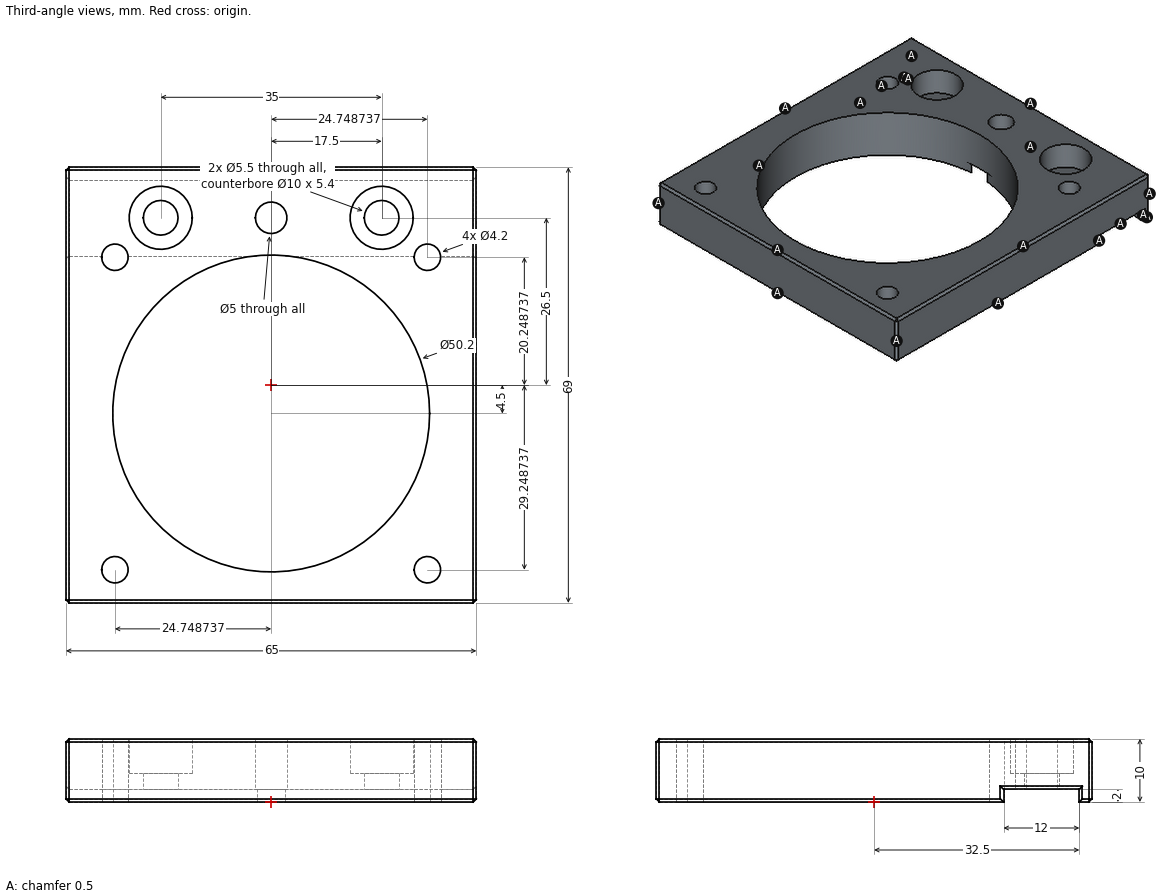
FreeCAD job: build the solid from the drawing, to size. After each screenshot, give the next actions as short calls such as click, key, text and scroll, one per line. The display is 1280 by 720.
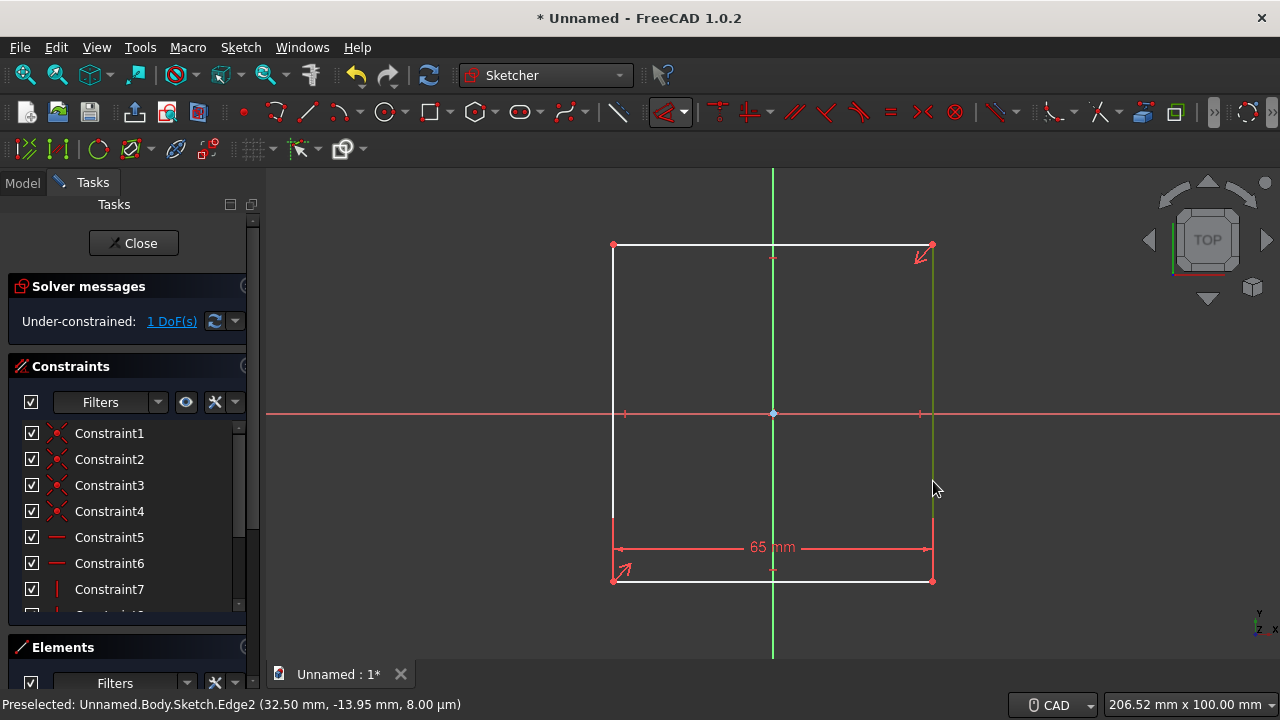
key(i)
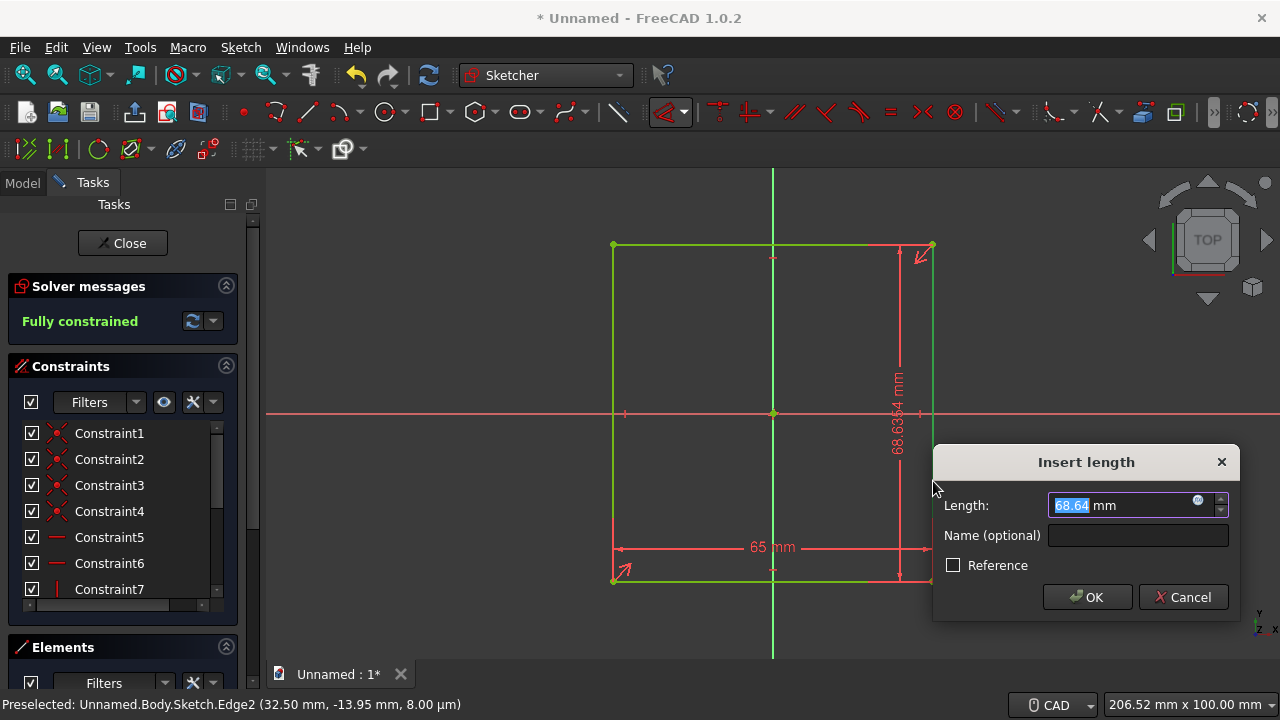
text(69)
key(Return)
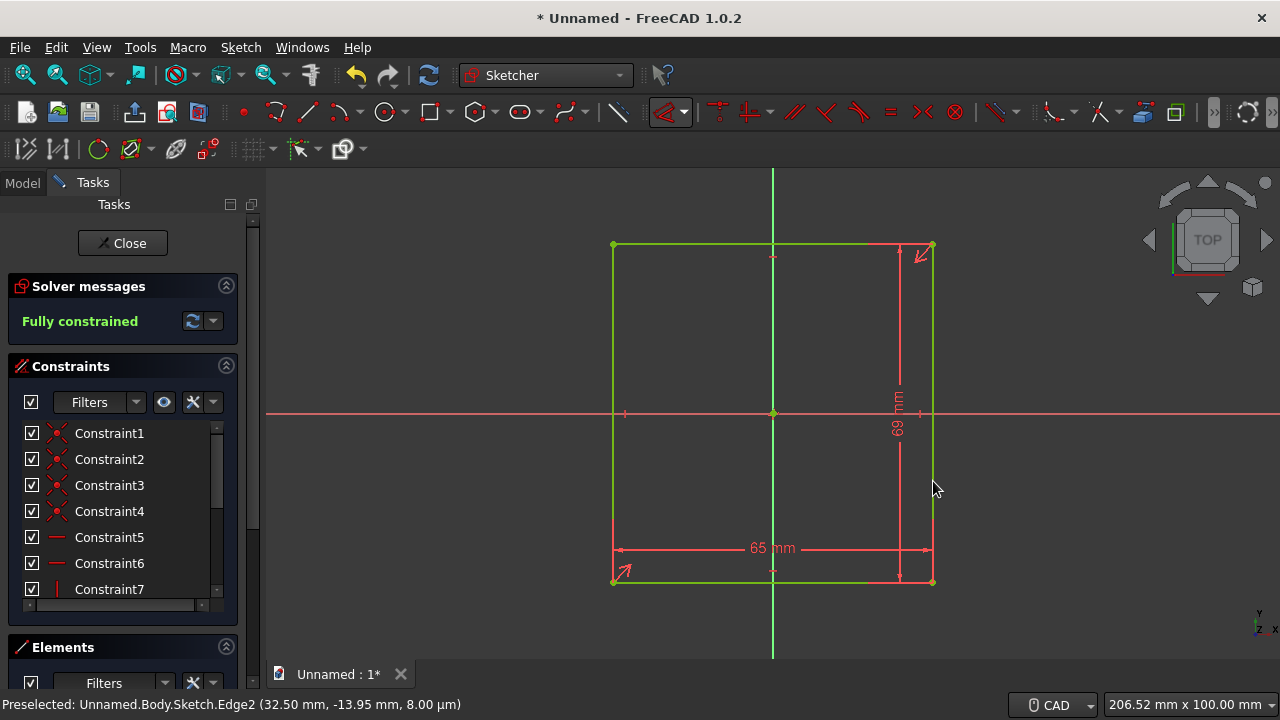
click(123, 243)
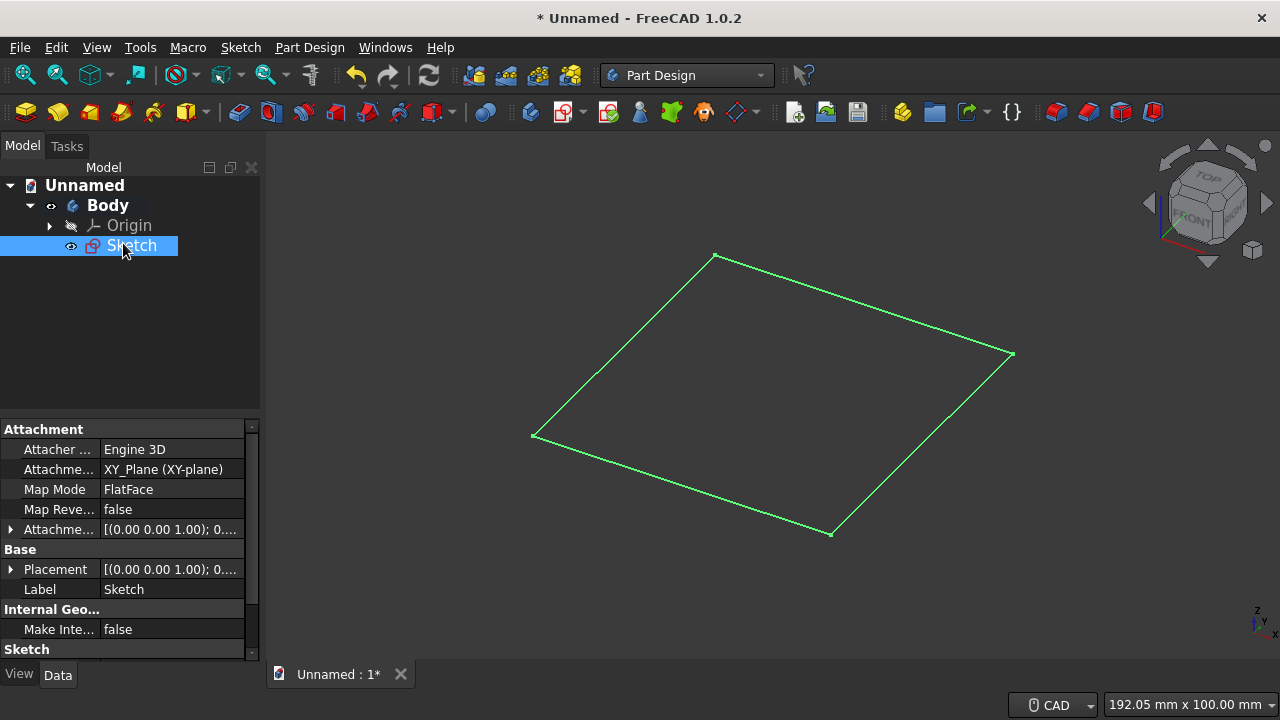
click(26, 112)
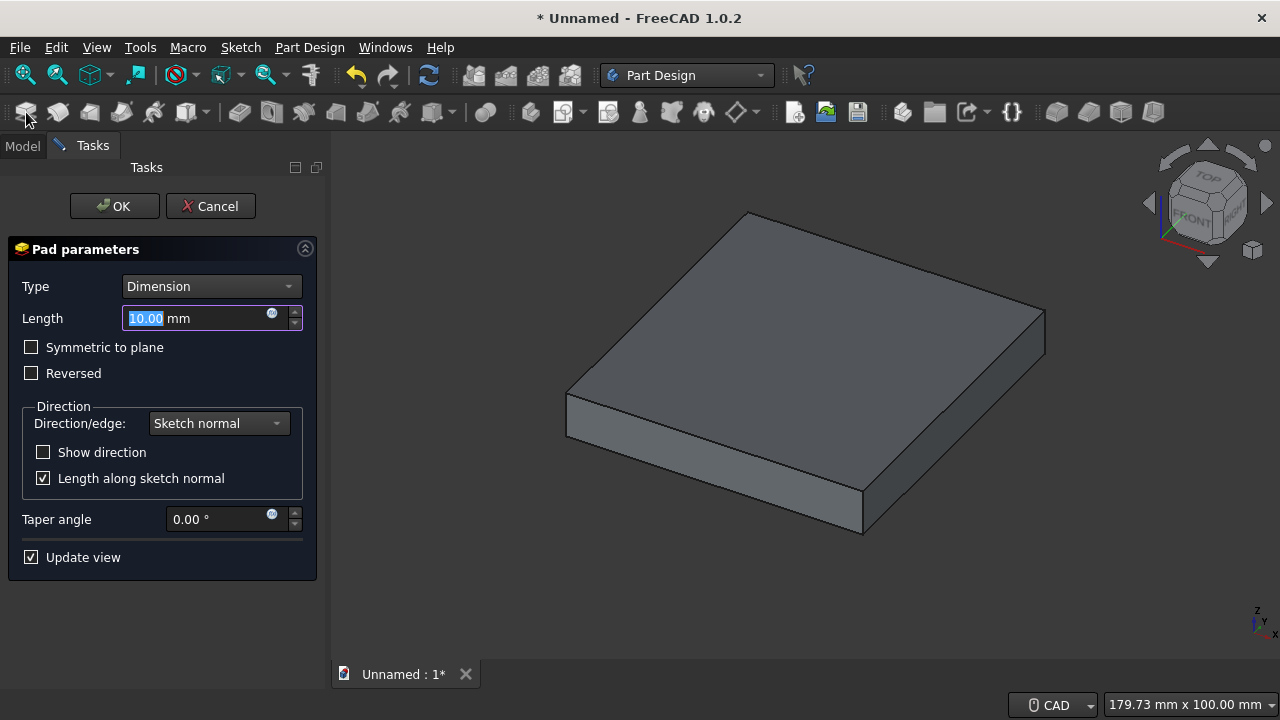
text(10)
key(Tab)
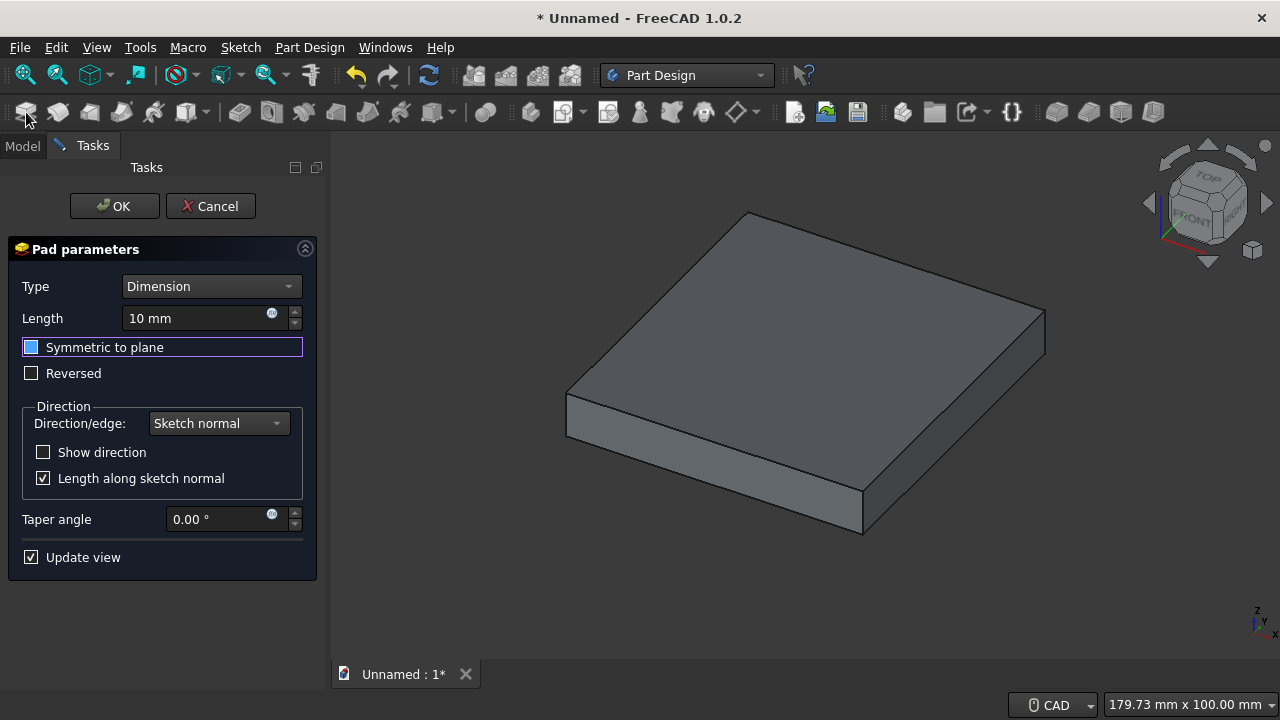
click(115, 206)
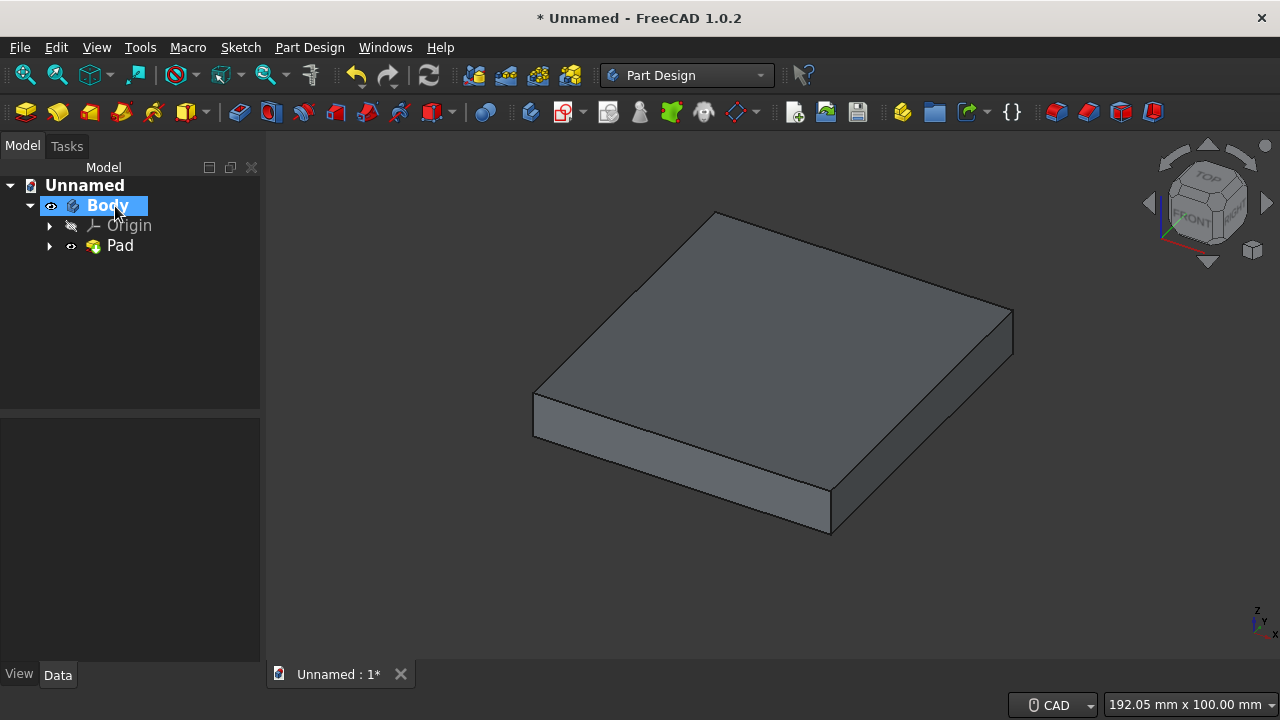
key(6)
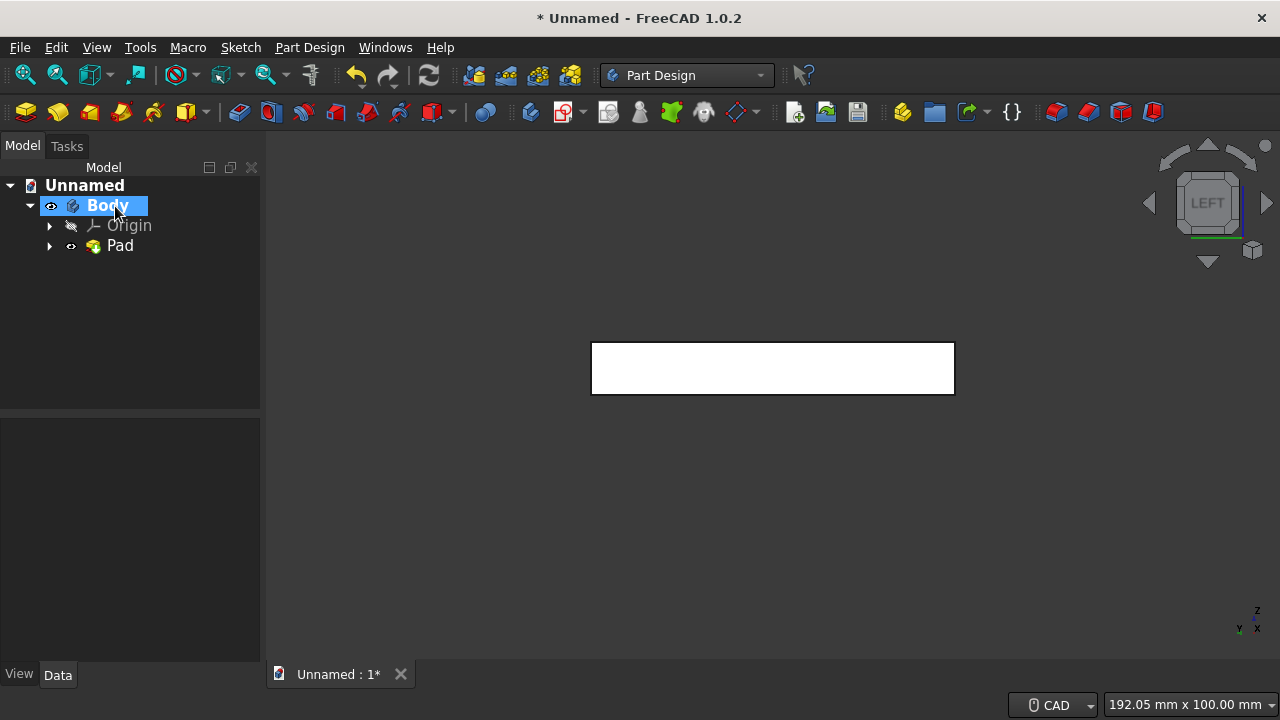
click(26, 76)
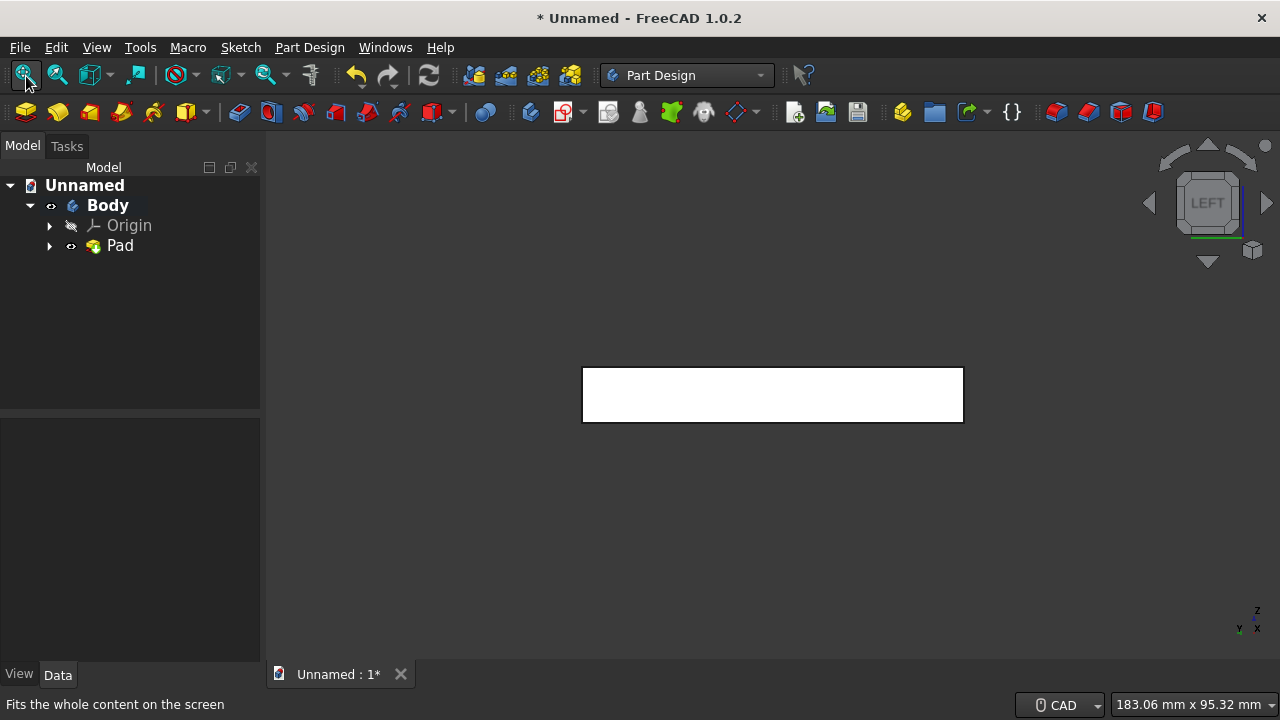
click(664, 394)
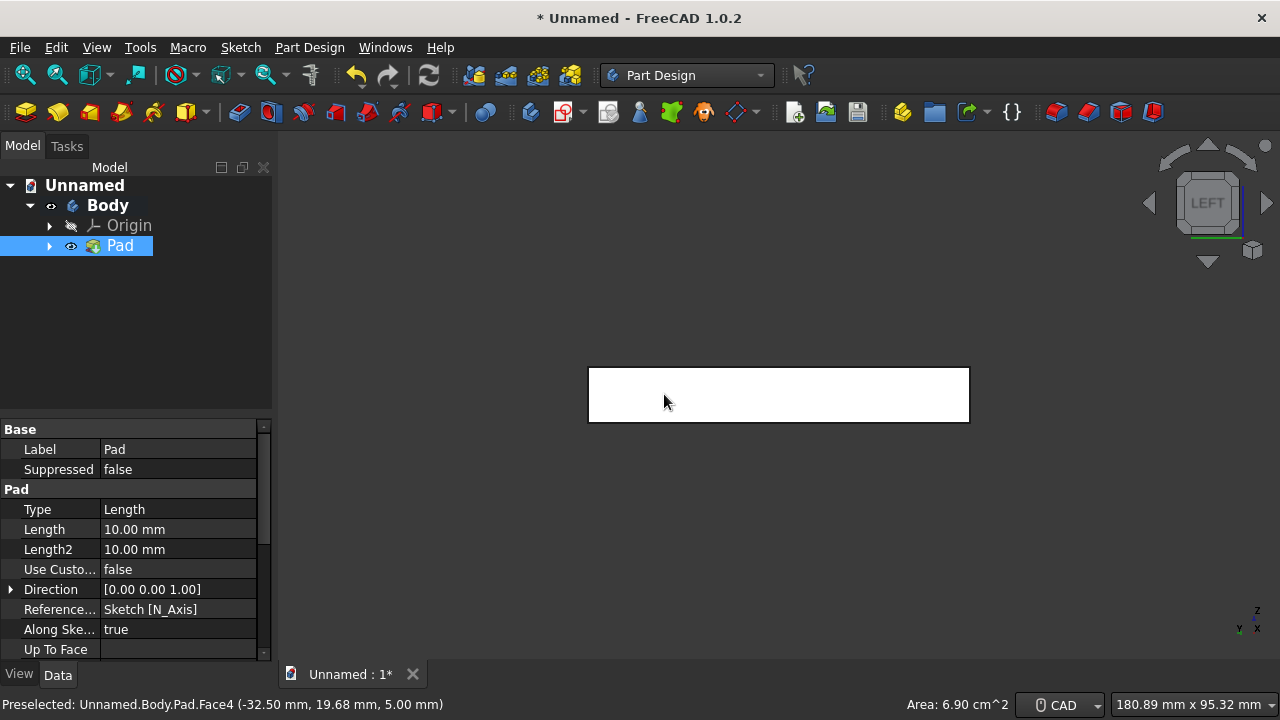
click(564, 112)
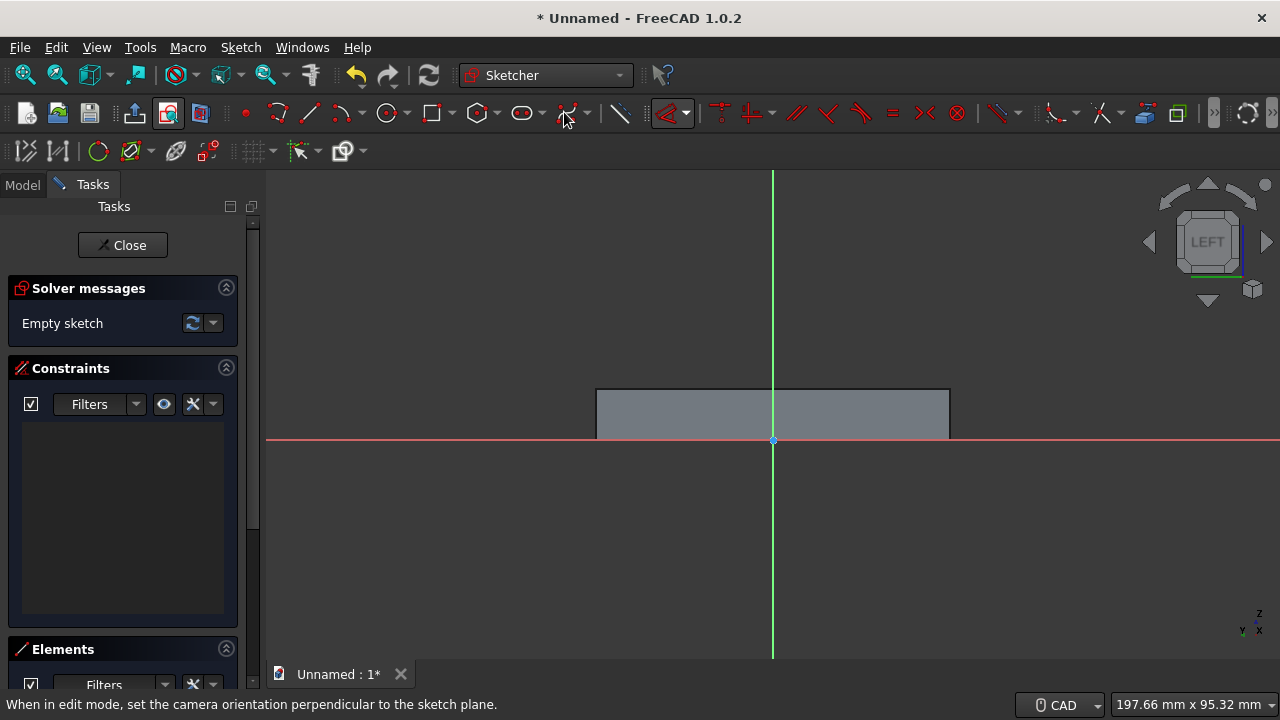
scroll(629, 438, up, 11)